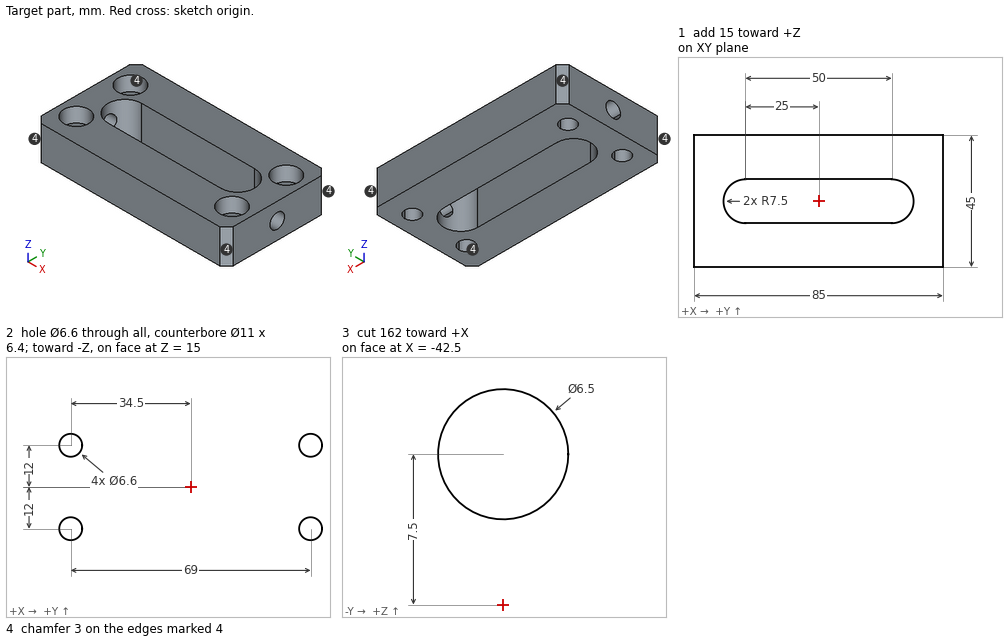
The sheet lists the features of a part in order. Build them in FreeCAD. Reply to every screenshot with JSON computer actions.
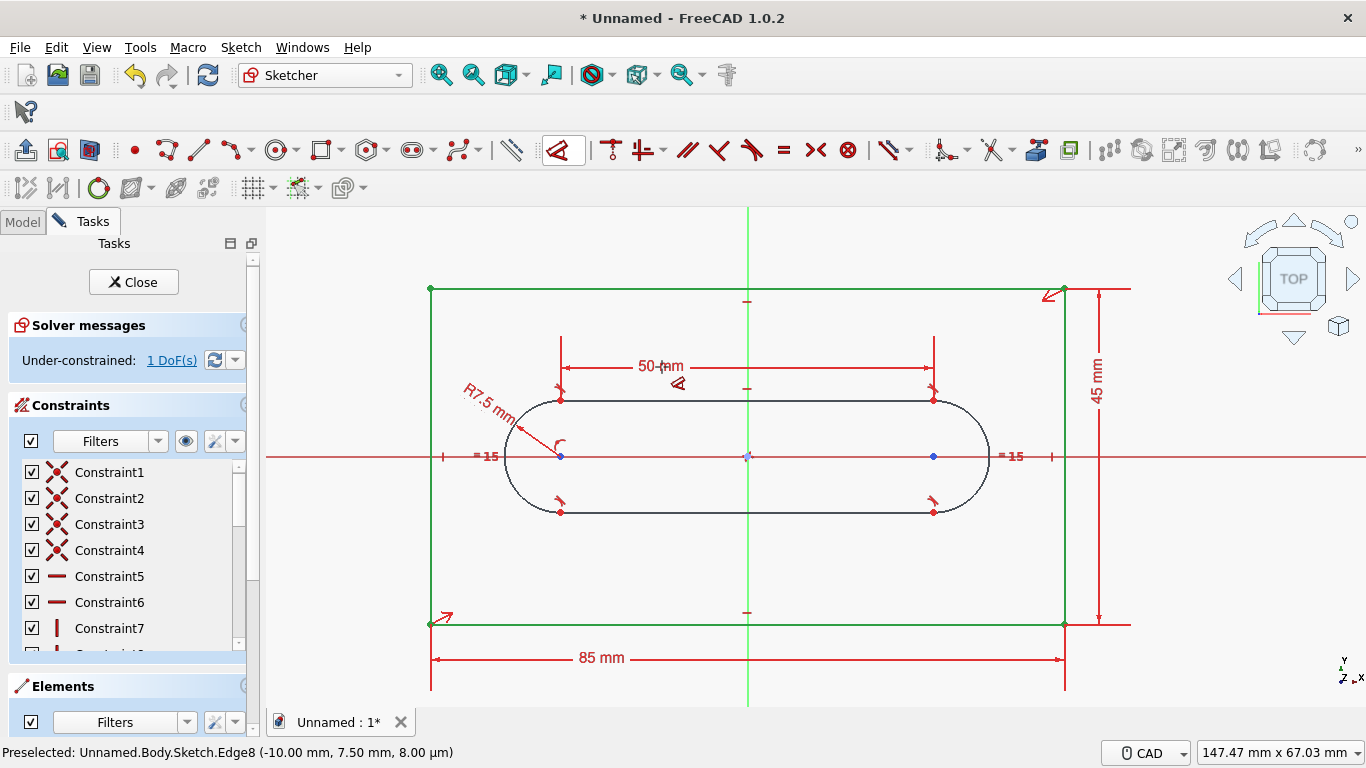
{"action": "left_click", "coordinate": [561, 401]}
{"action": "left_click", "coordinate": [589, 367]}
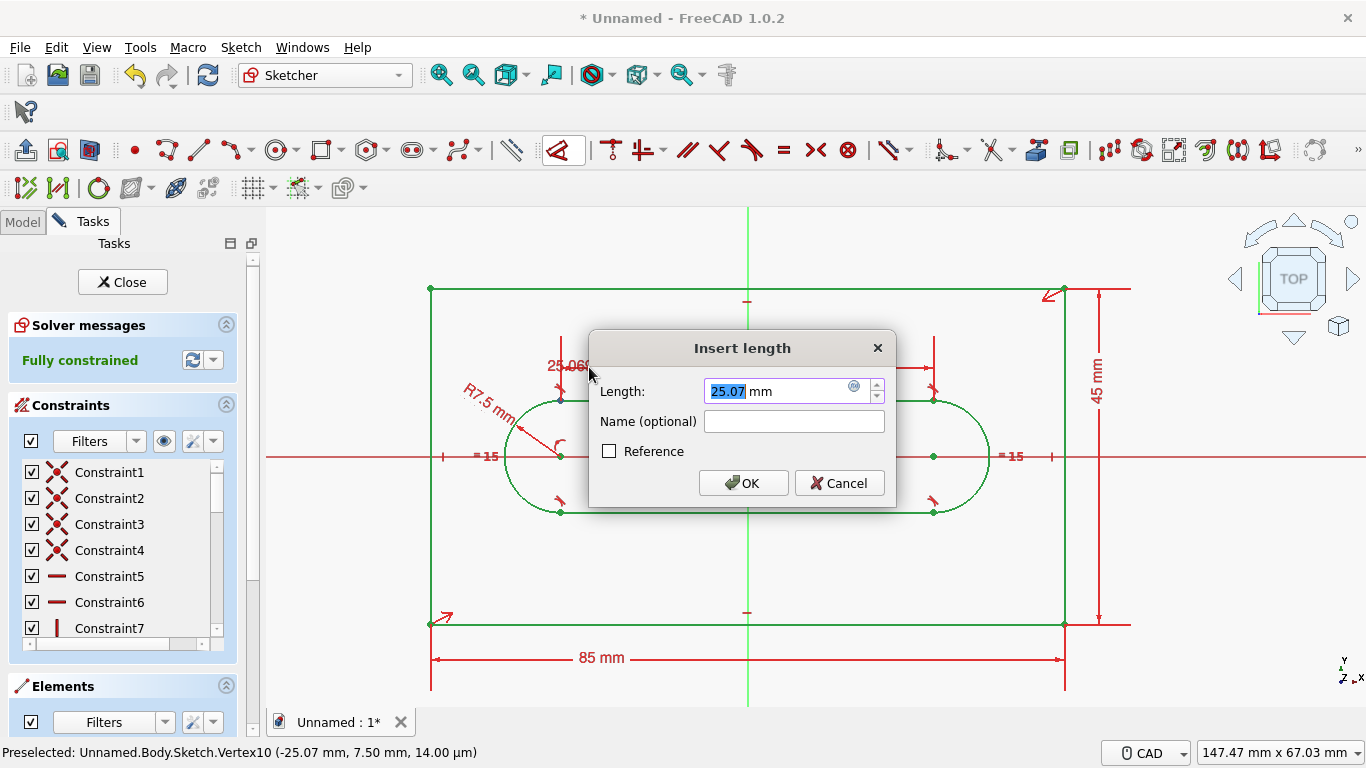
{"action": "type", "text": "25"}
{"action": "key", "text": "Return"}
{"action": "key", "text": "Escape"}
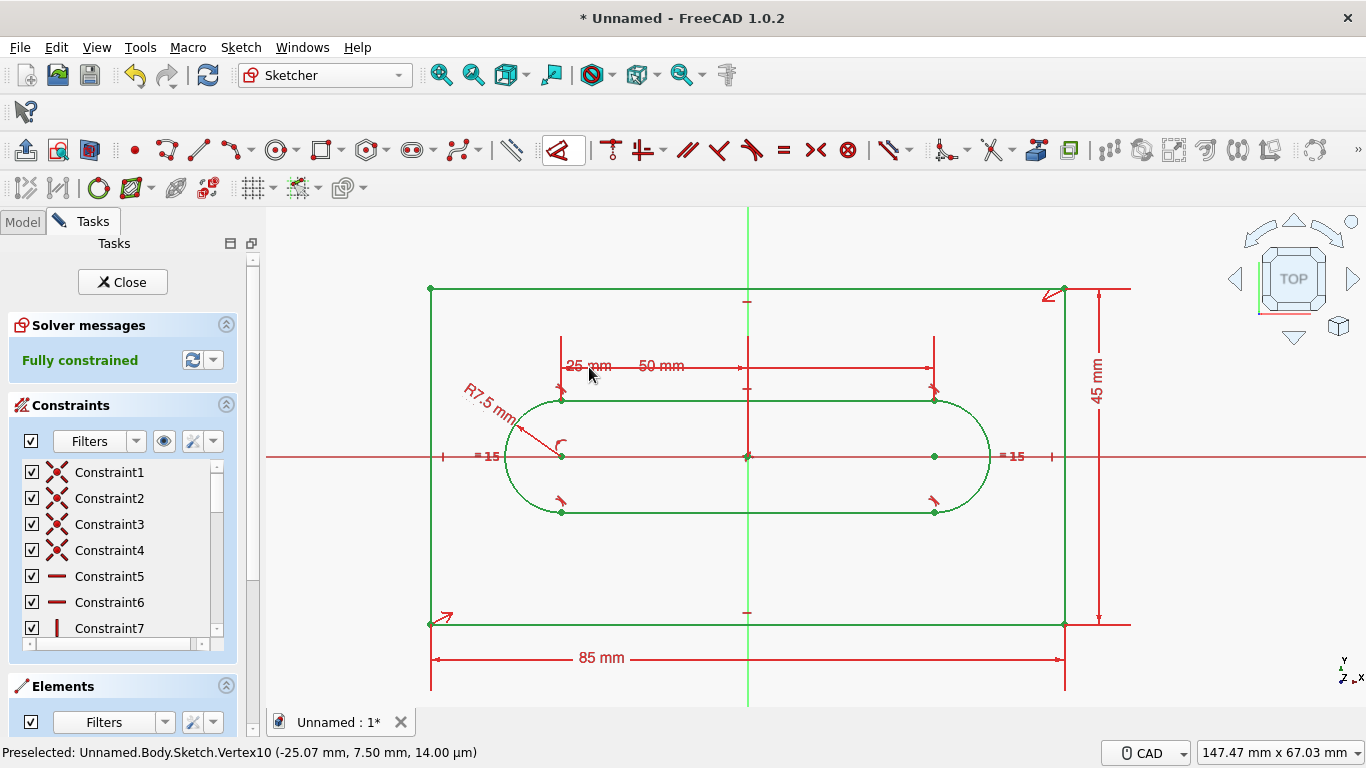
{"action": "left_click", "coordinate": [123, 282]}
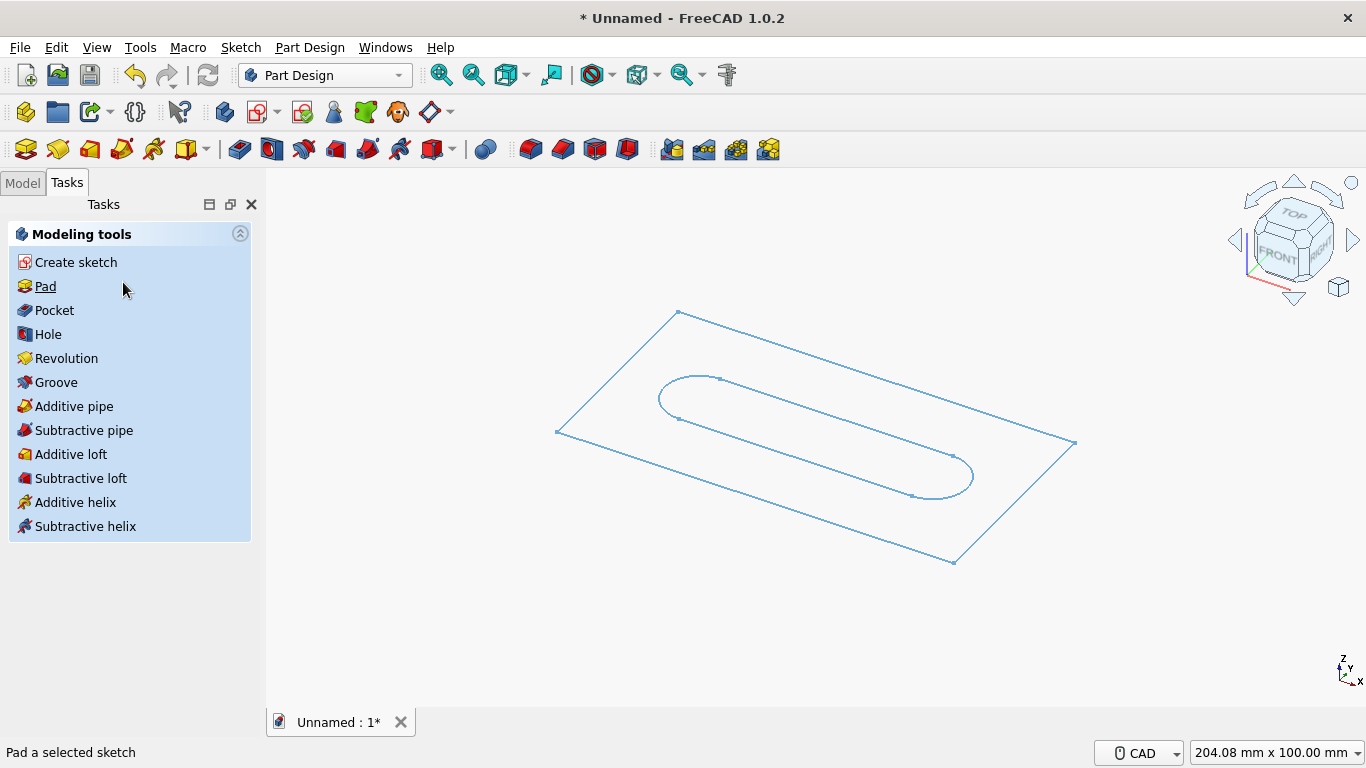
{"action": "left_click", "coordinate": [26, 150]}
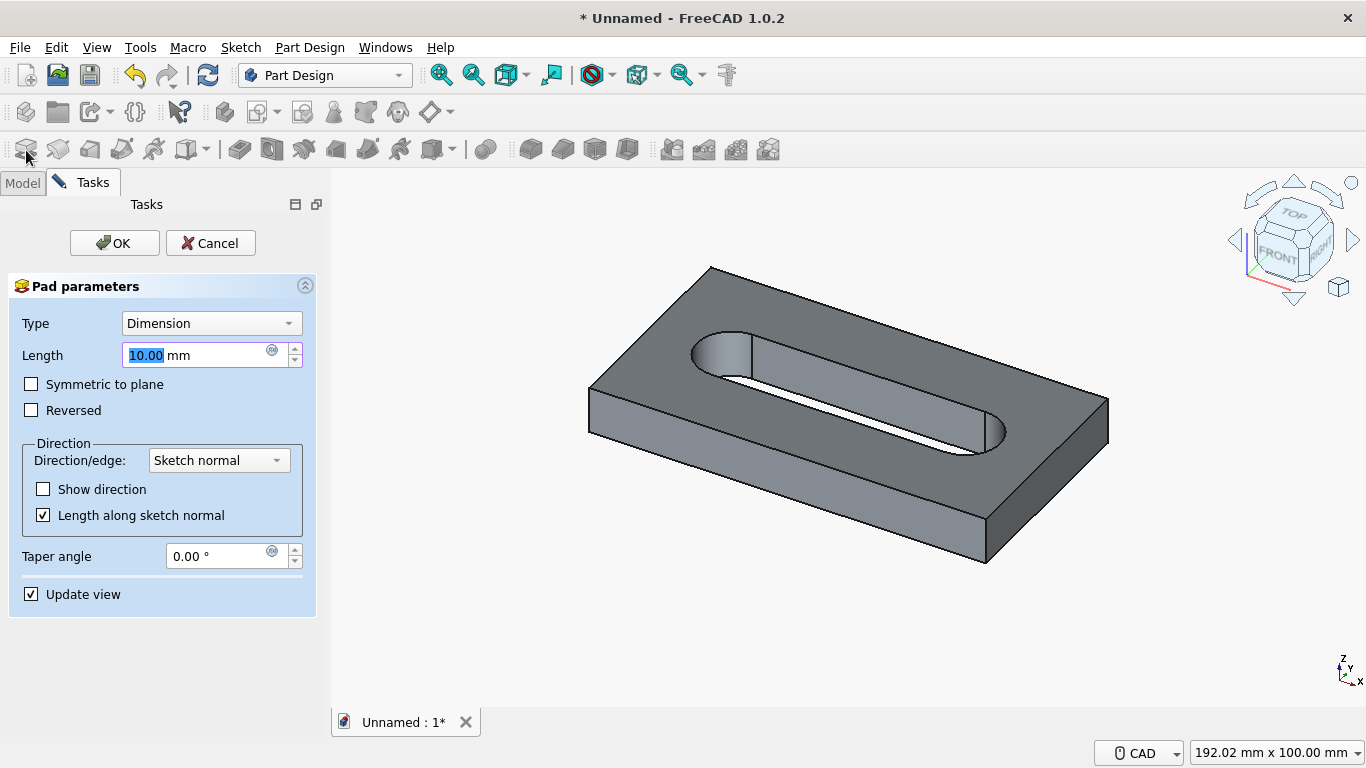
{"action": "type", "text": "15"}
{"action": "key", "text": "Tab"}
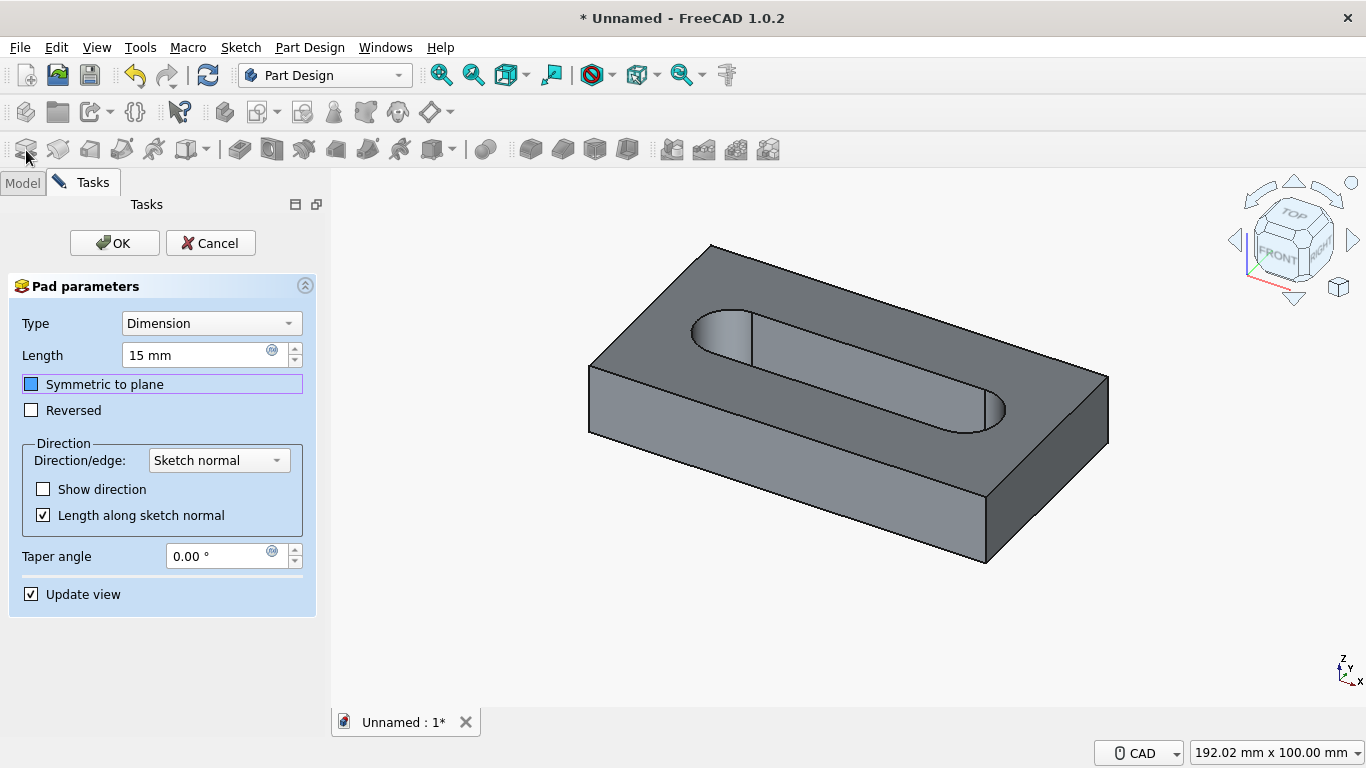
{"action": "left_click", "coordinate": [115, 243]}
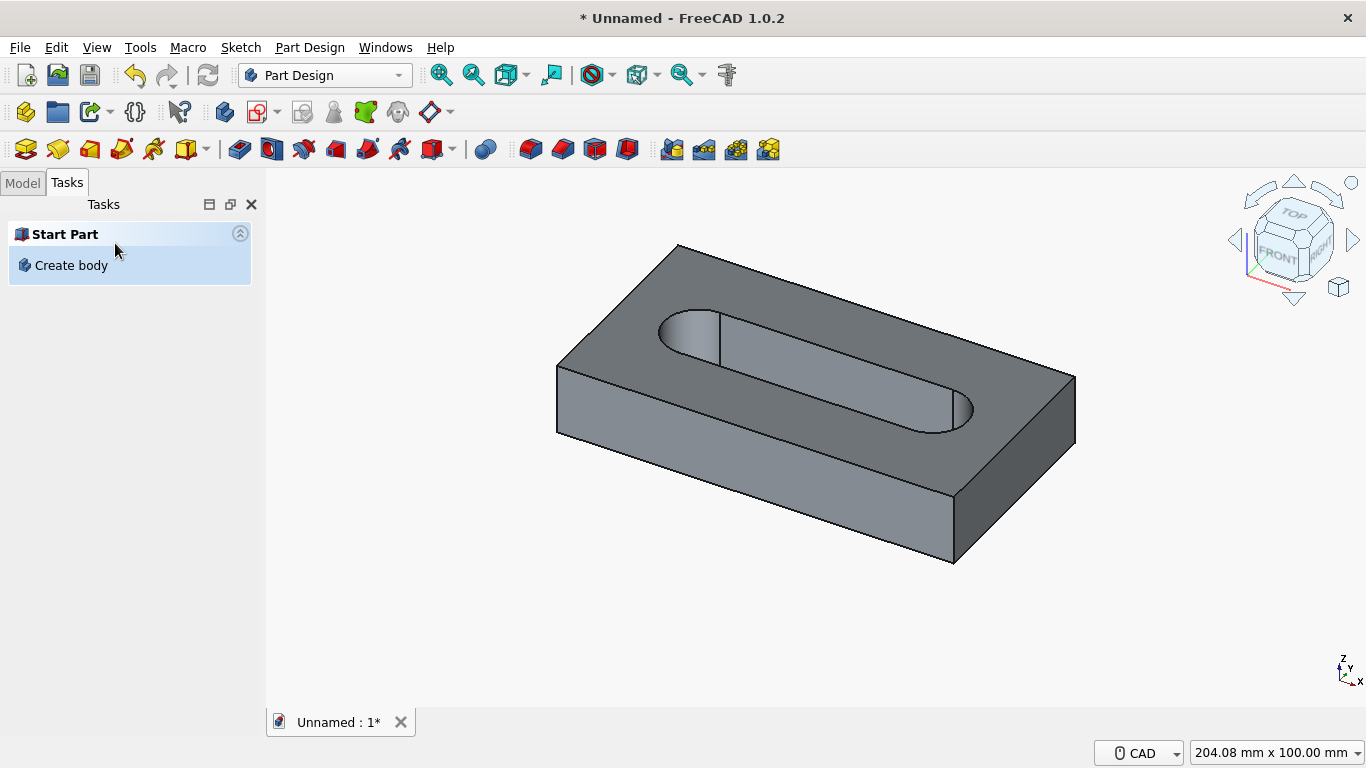
{"action": "left_click", "coordinate": [1021, 392]}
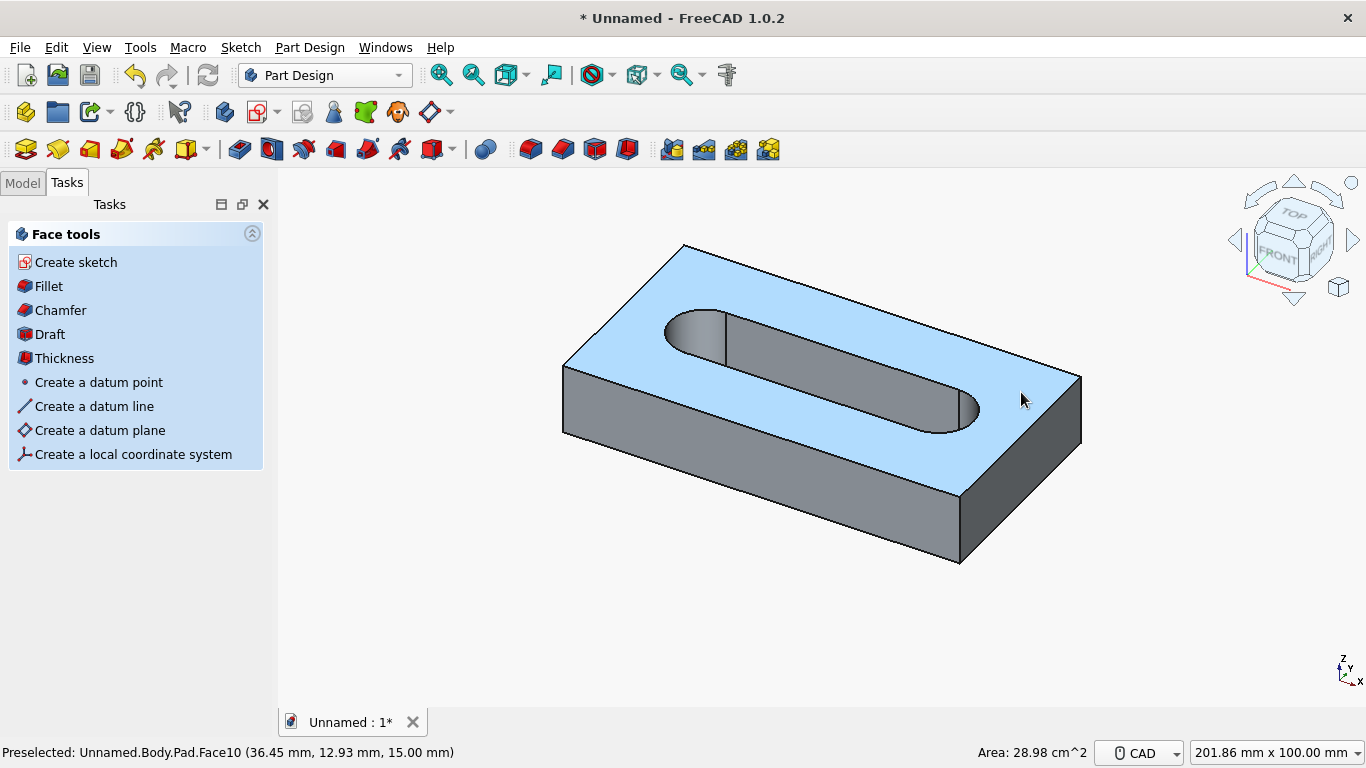
{"action": "left_click", "coordinate": [258, 112]}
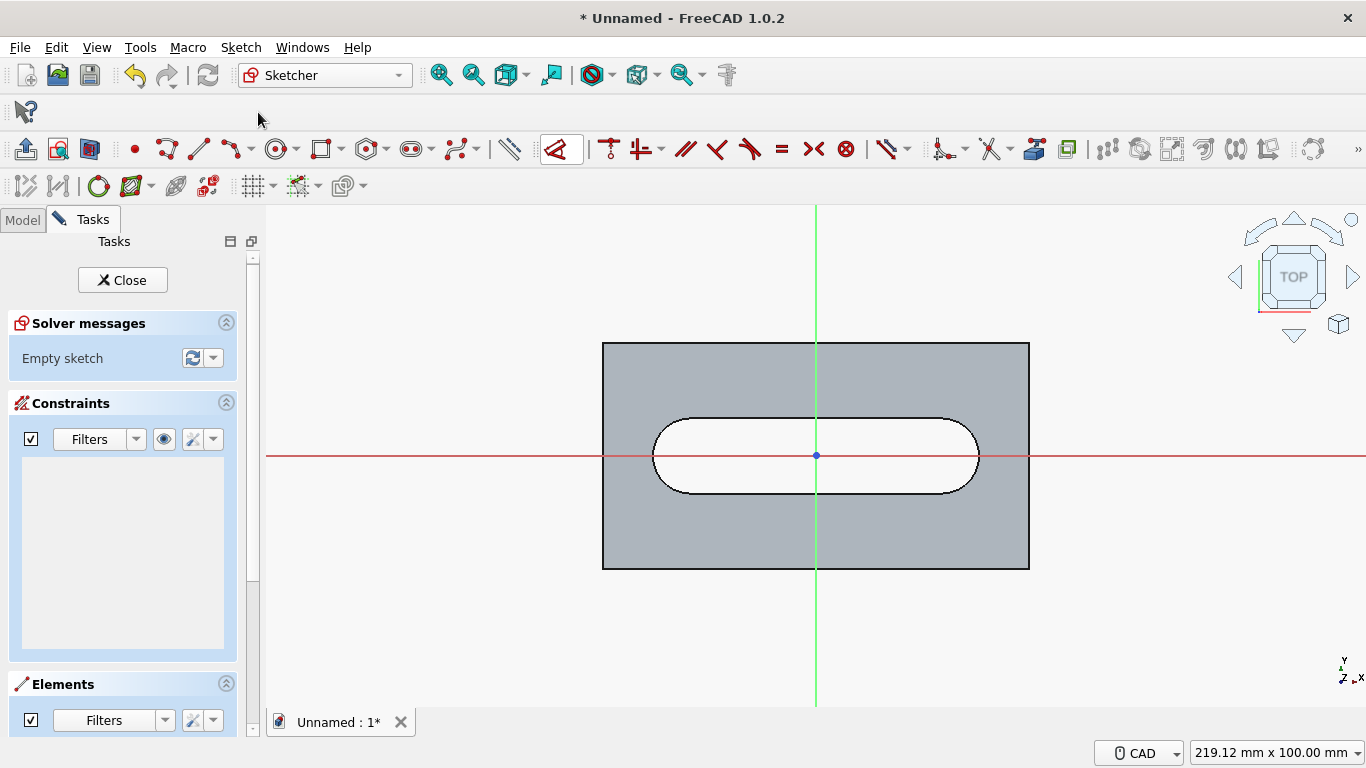
{"action": "scroll", "coordinate": [899, 456], "scroll_direction": "up", "scroll_amount": 3}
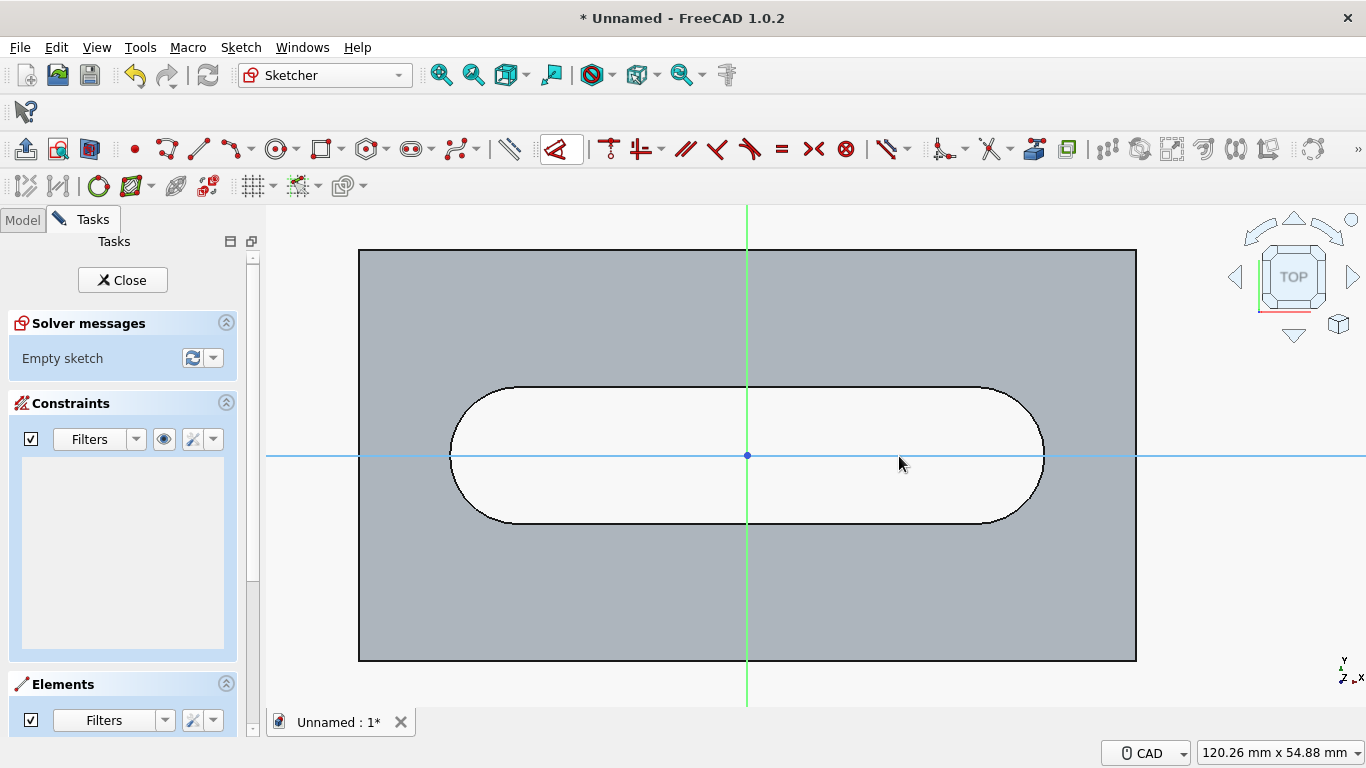
{"action": "key", "text": "g c"}